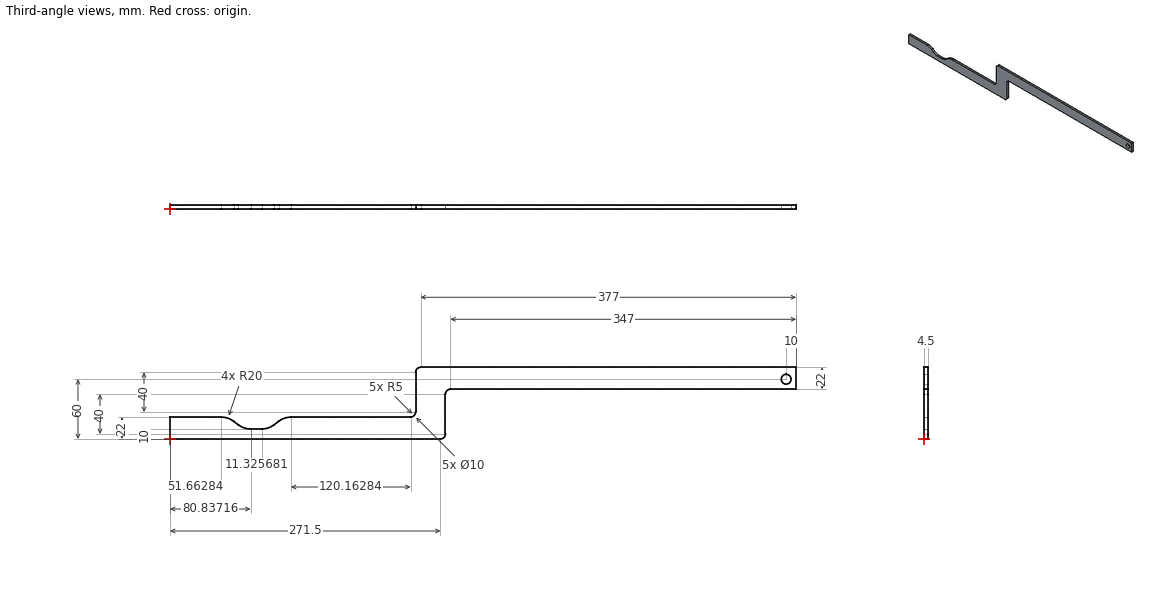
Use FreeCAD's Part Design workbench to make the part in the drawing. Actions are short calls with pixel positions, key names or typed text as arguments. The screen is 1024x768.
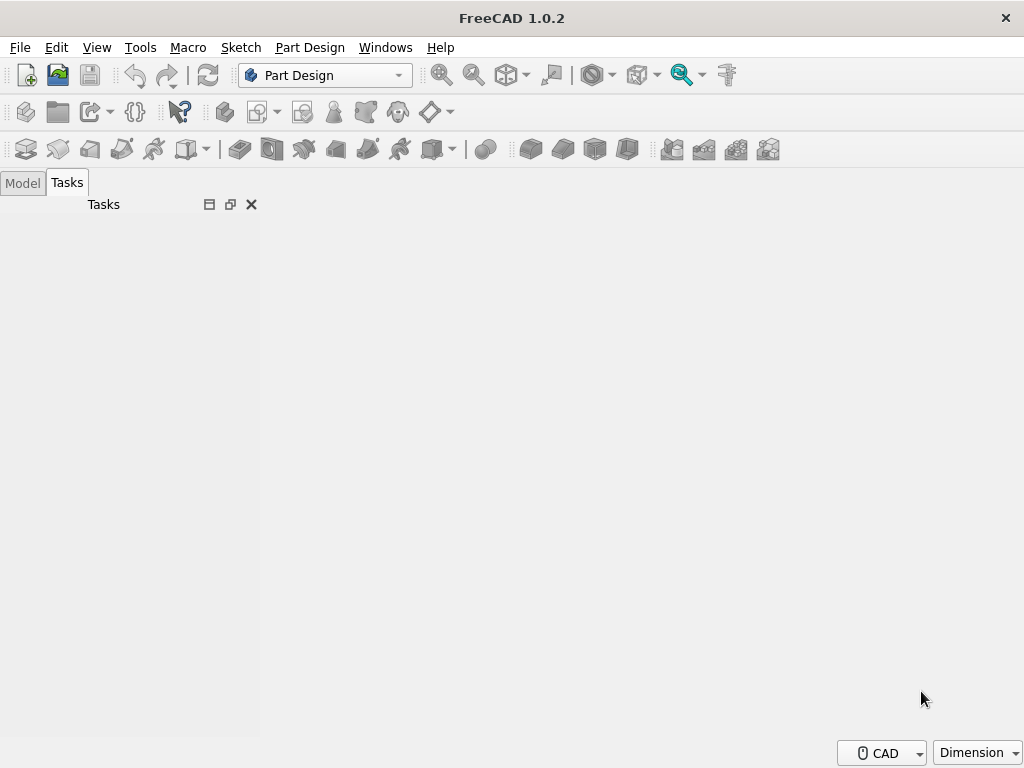
key(ctrl+n)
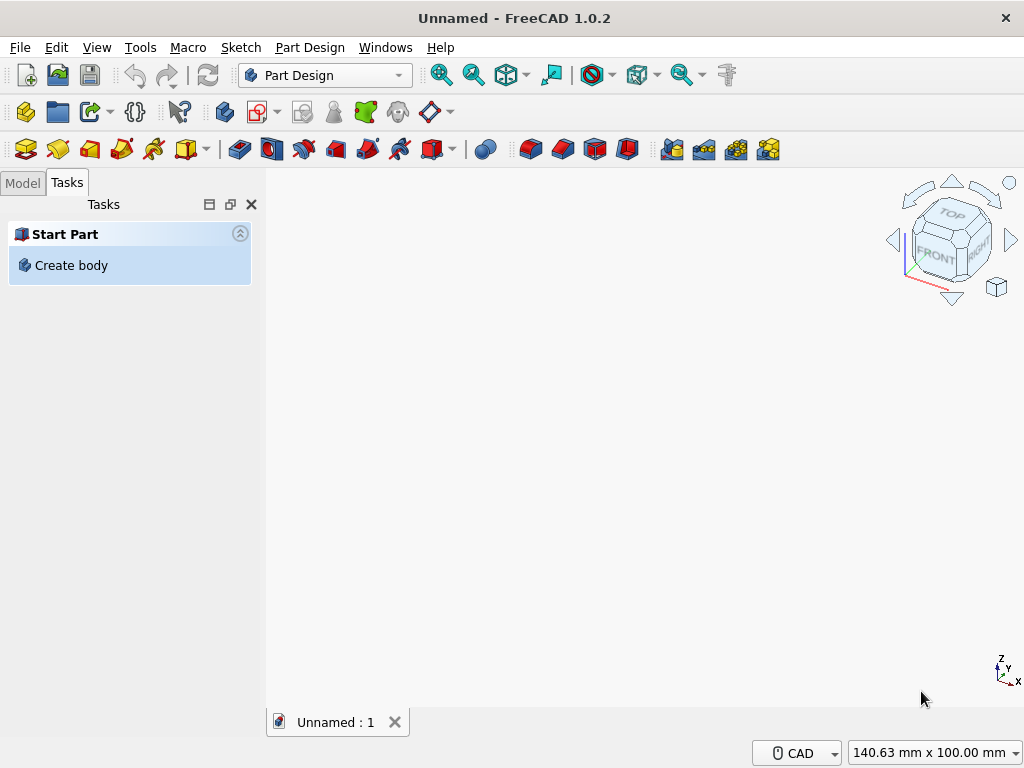
click(258, 112)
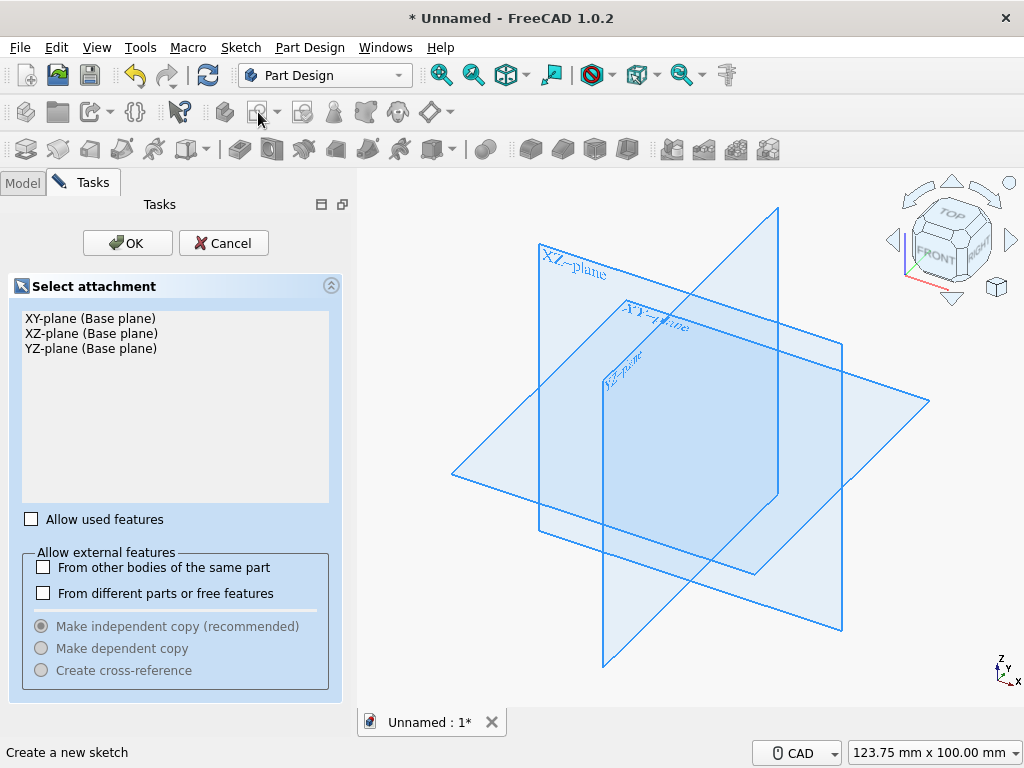
click(82, 334)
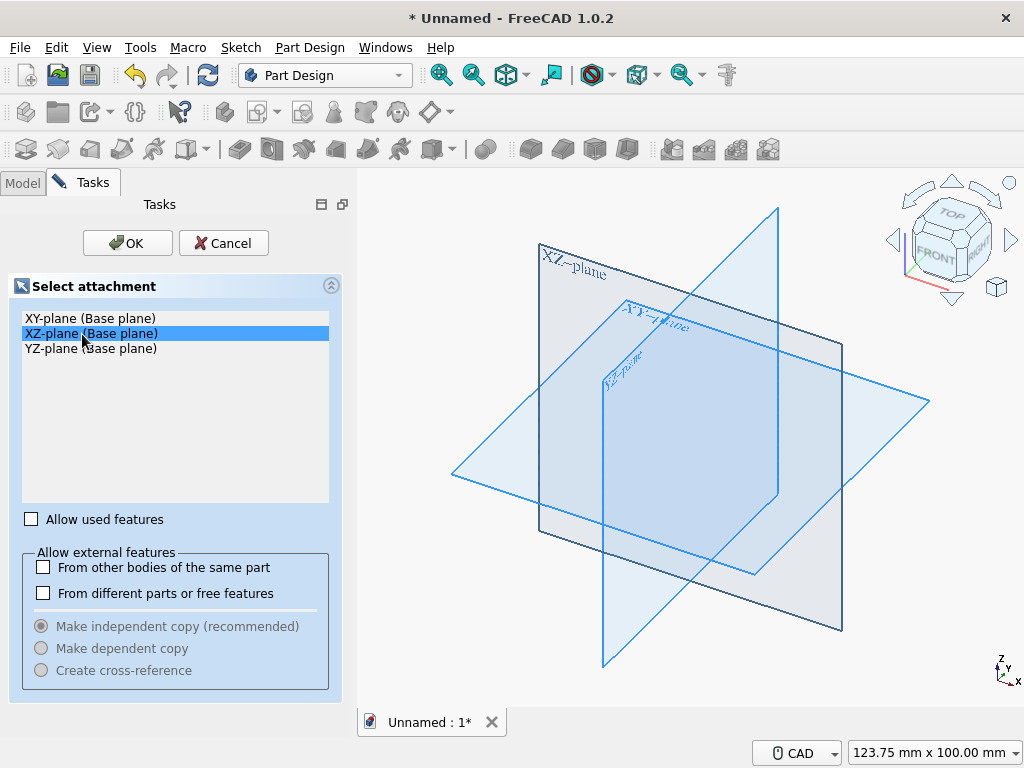
click(128, 243)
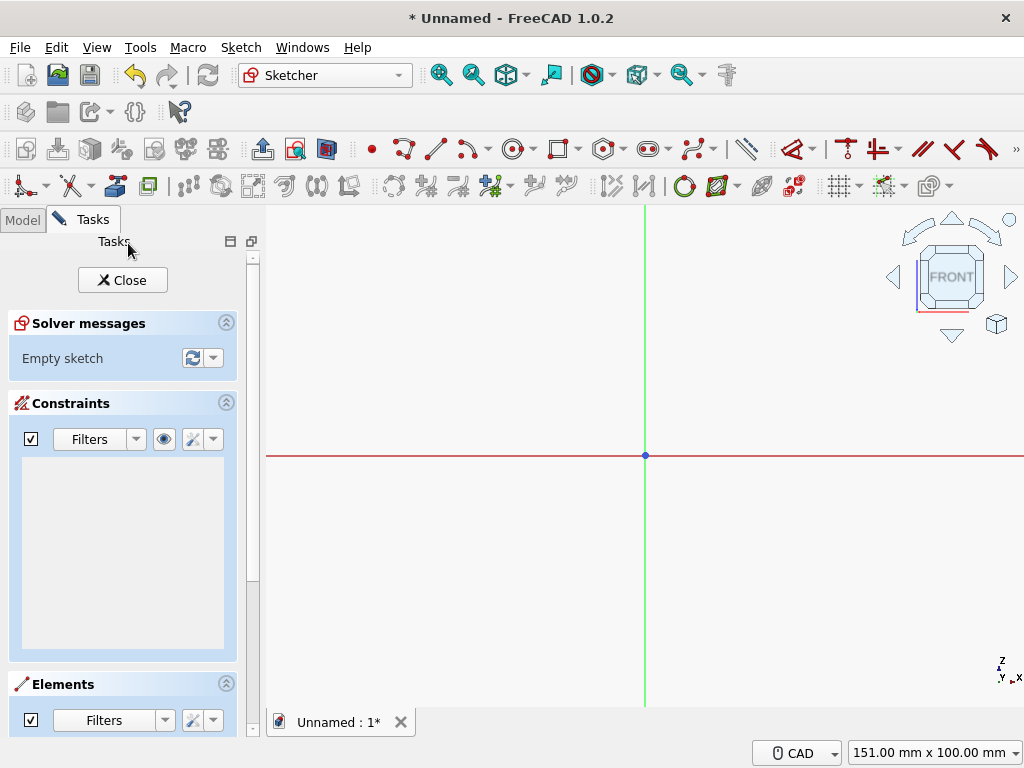
scroll(319, 484, down, 10)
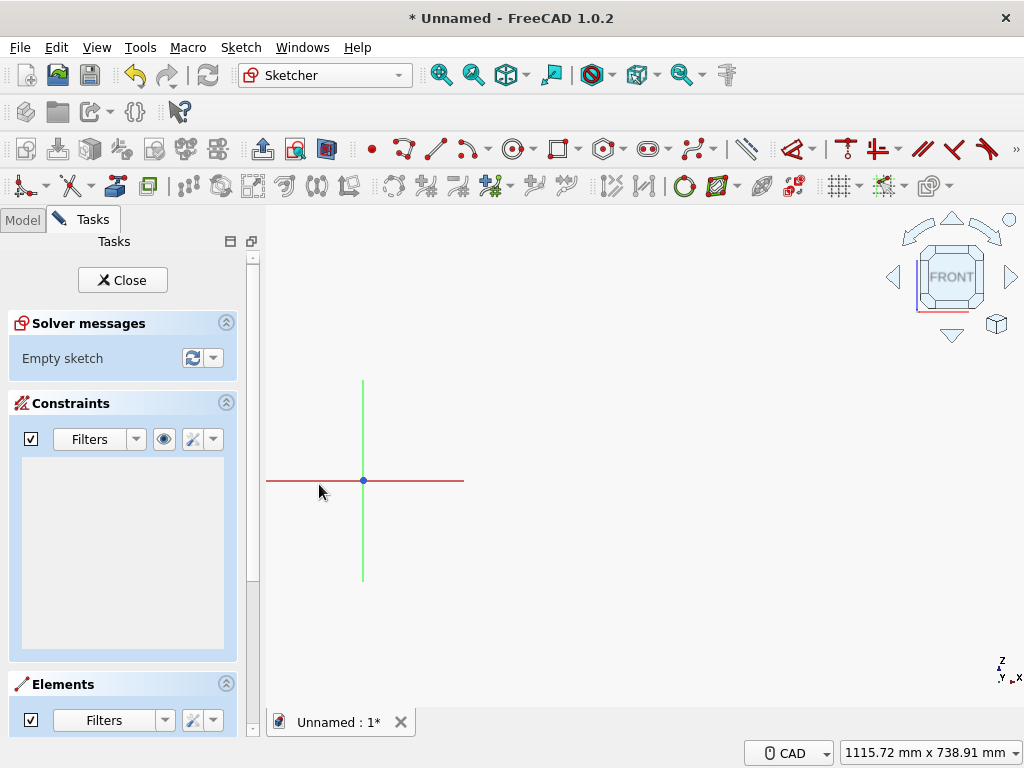
key(g)
key(m)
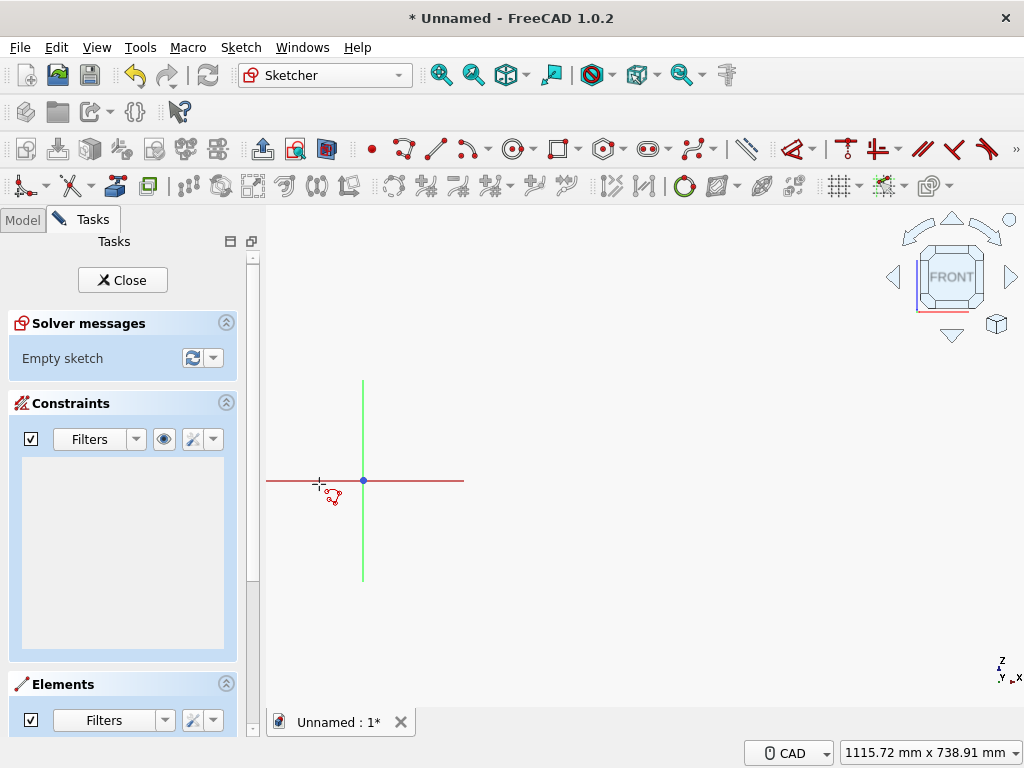
click(548, 481)
click(363, 481)
click(372, 466)
click(398, 466)
right_click(398, 466)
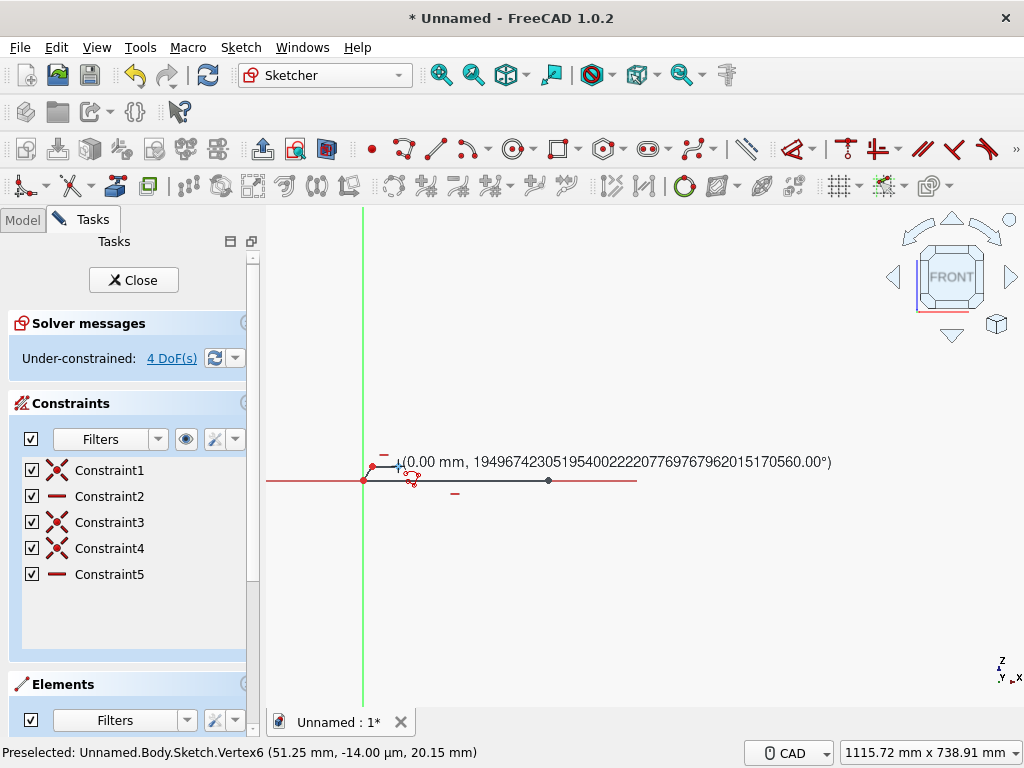
click(436, 150)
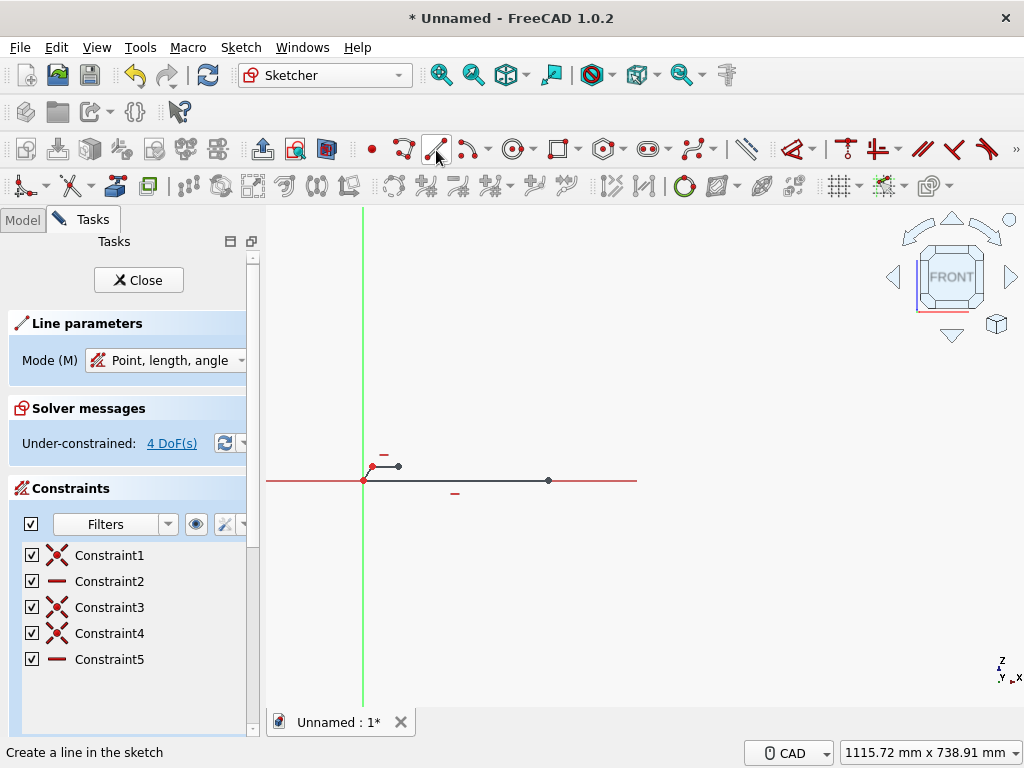
scroll(407, 469, up, 3)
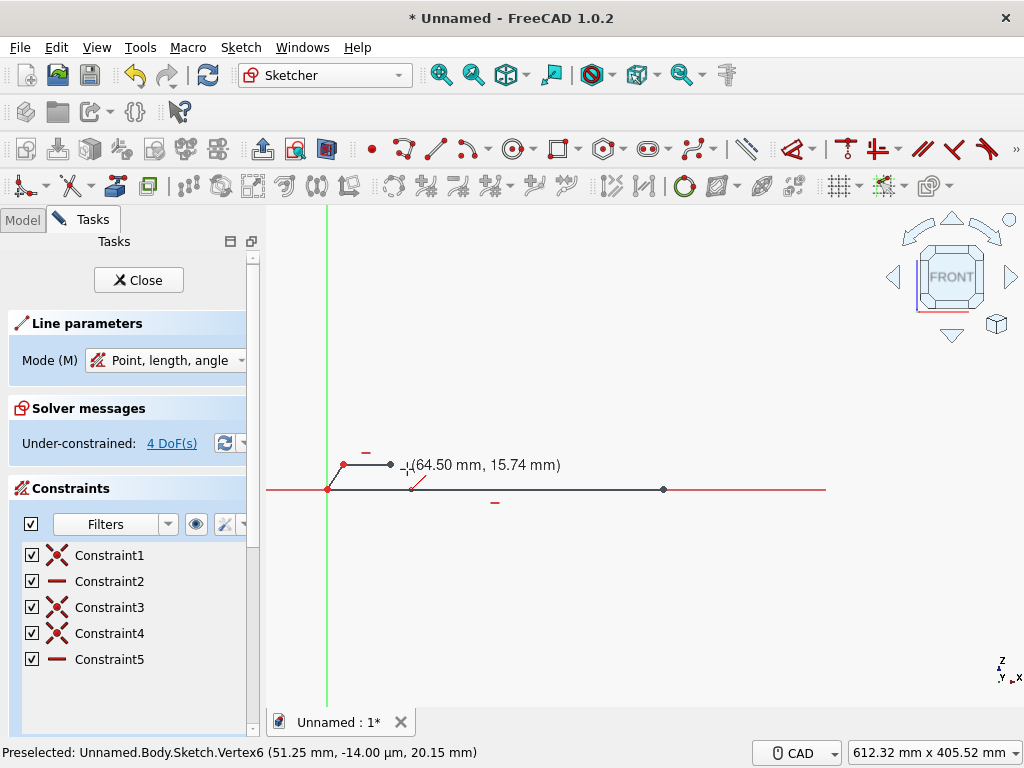
click(406, 468)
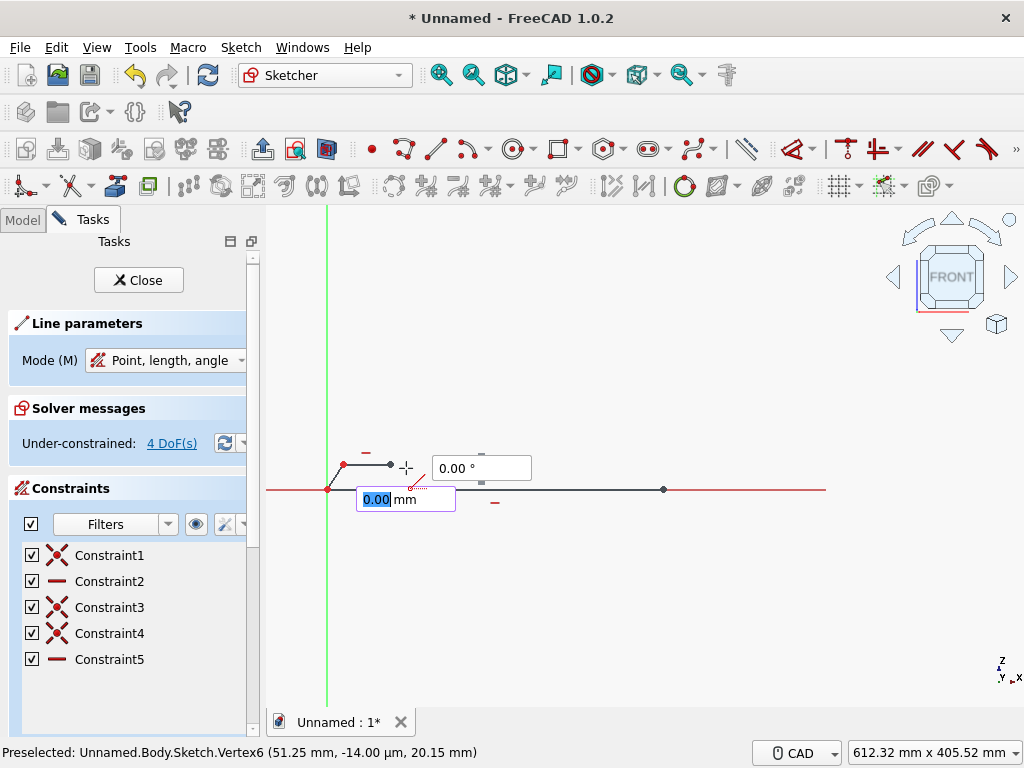
scroll(412, 472, up, 4)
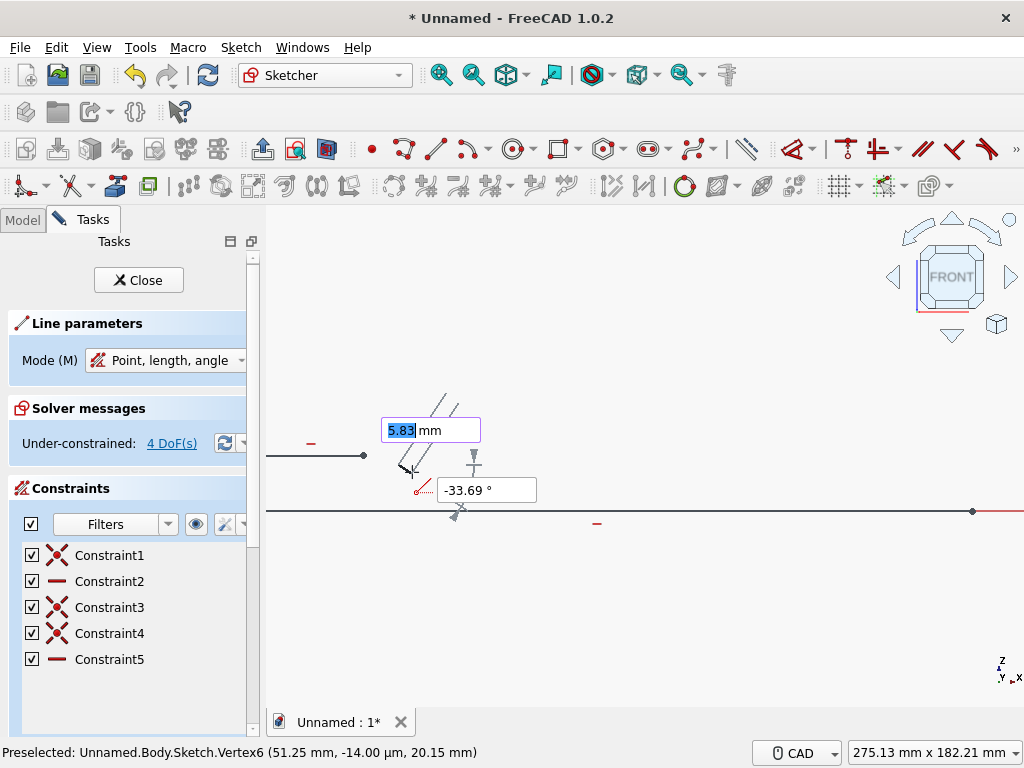
click(412, 472)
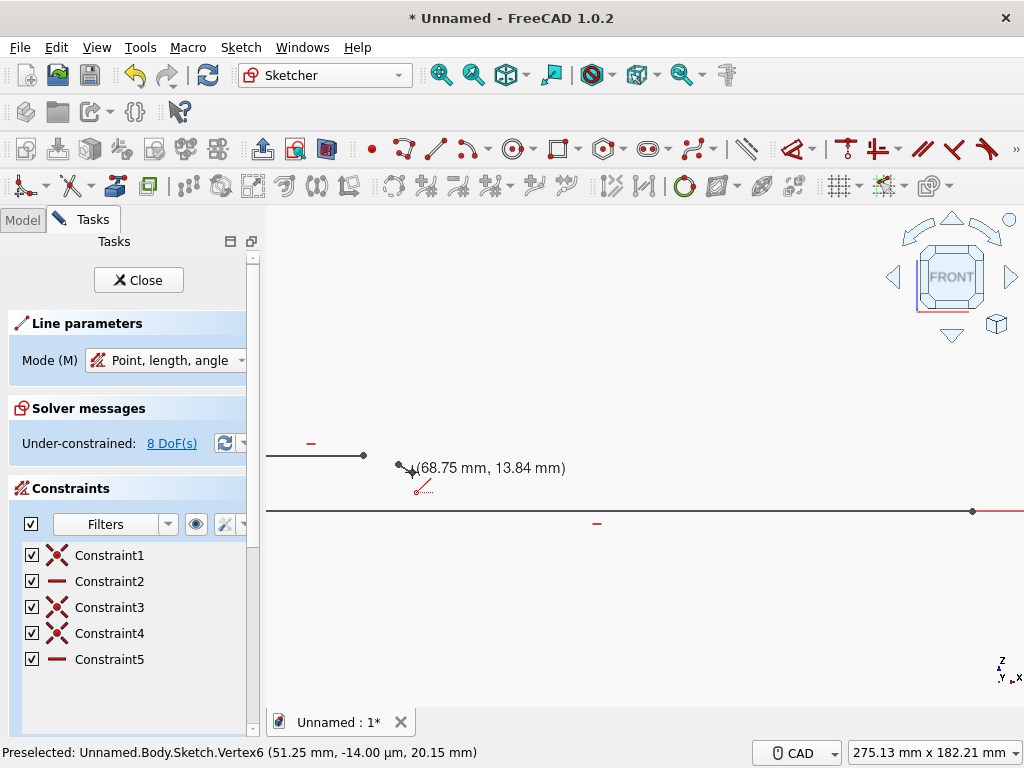
click(445, 484)
click(477, 484)